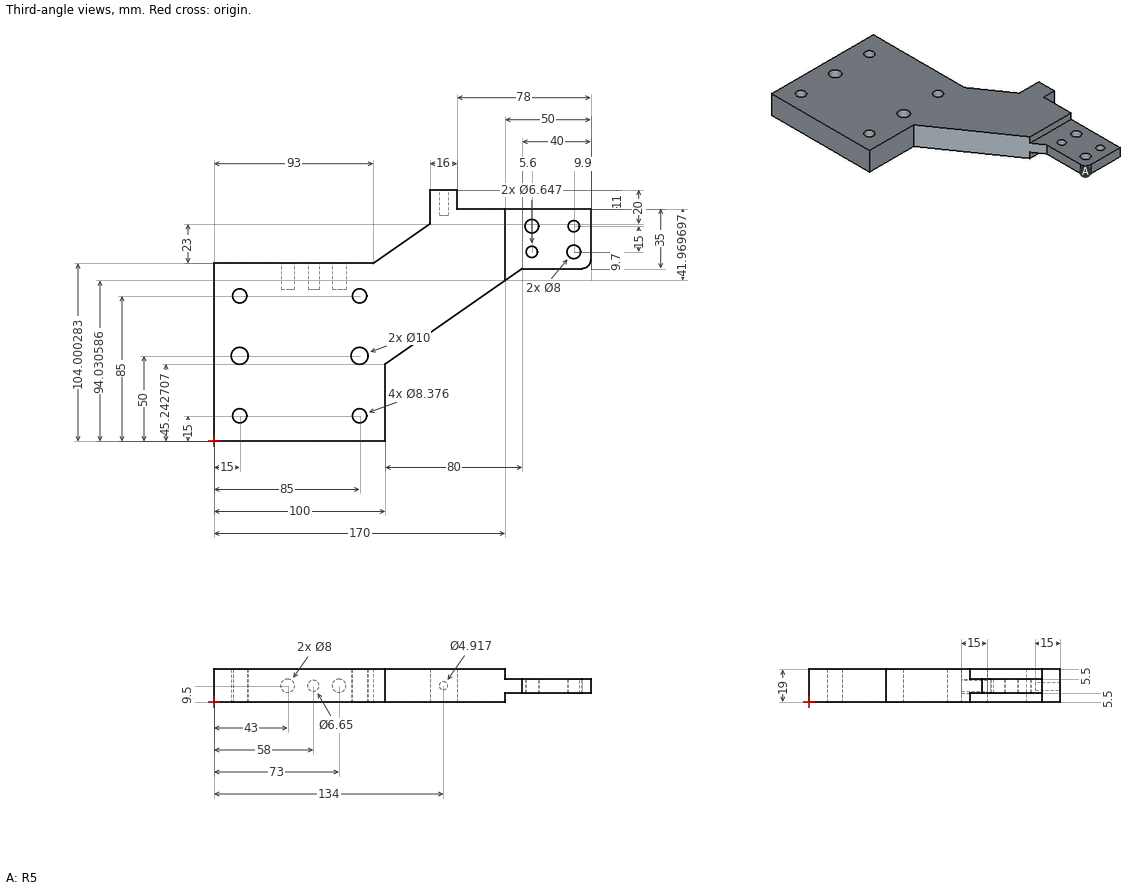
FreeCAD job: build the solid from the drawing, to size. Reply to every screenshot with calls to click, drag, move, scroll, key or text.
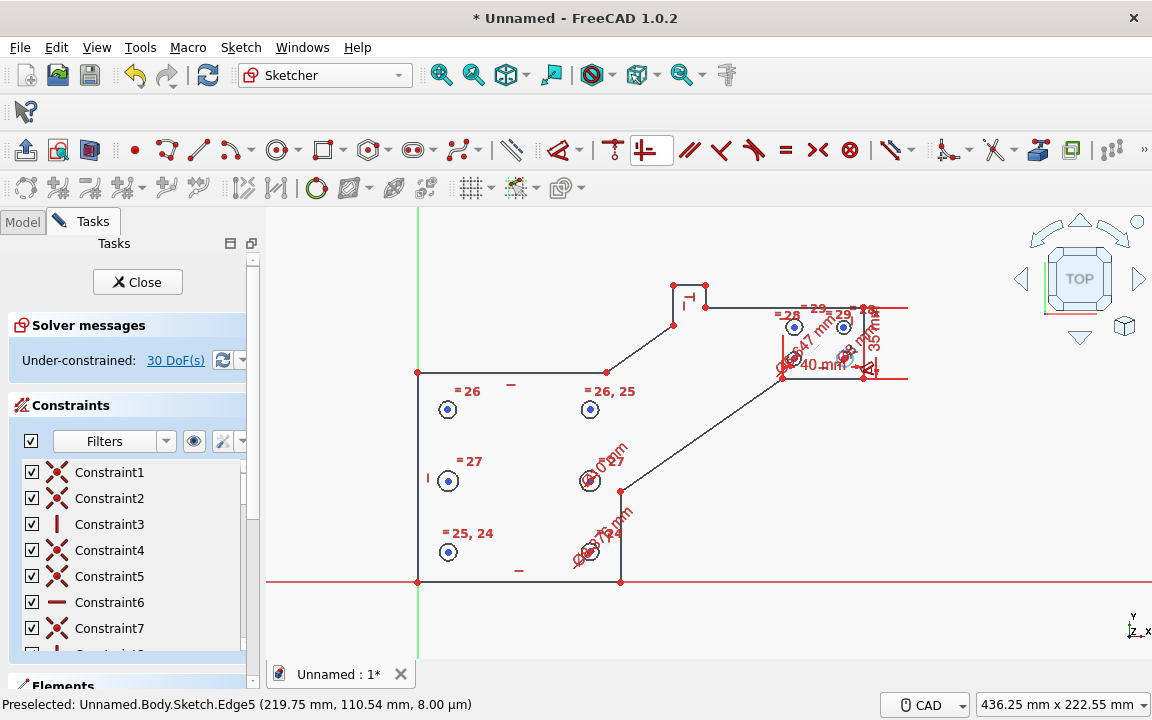
click(816, 308)
click(785, 274)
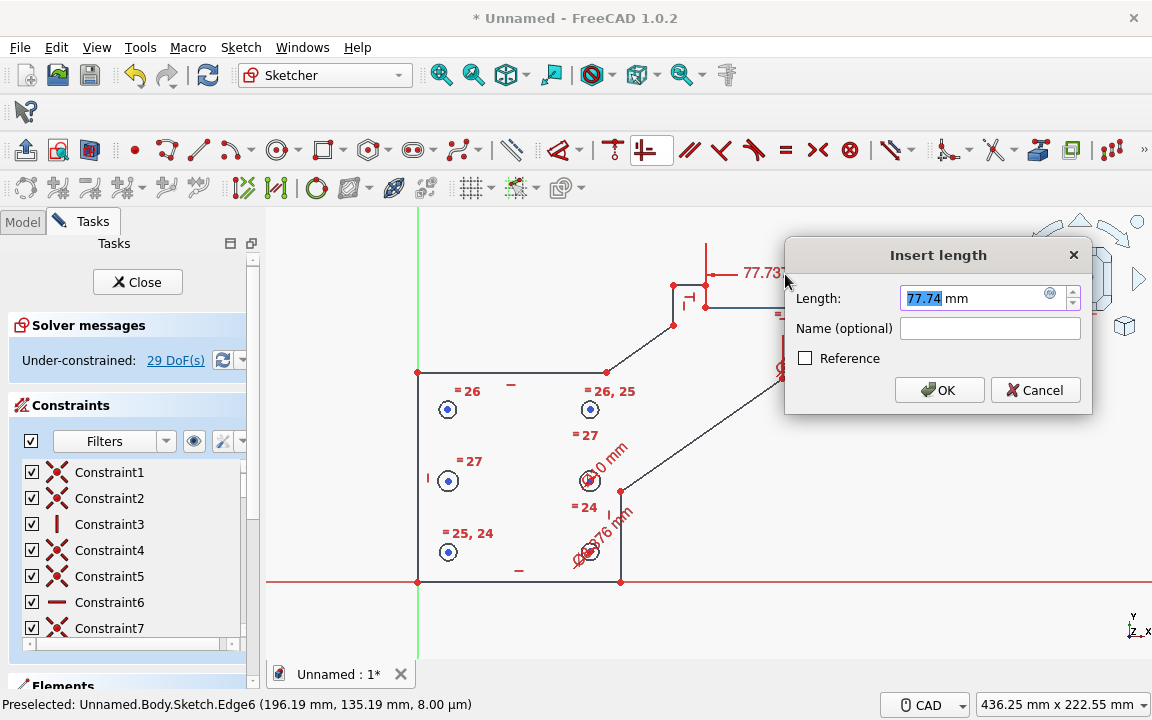
text(78)
key(Return)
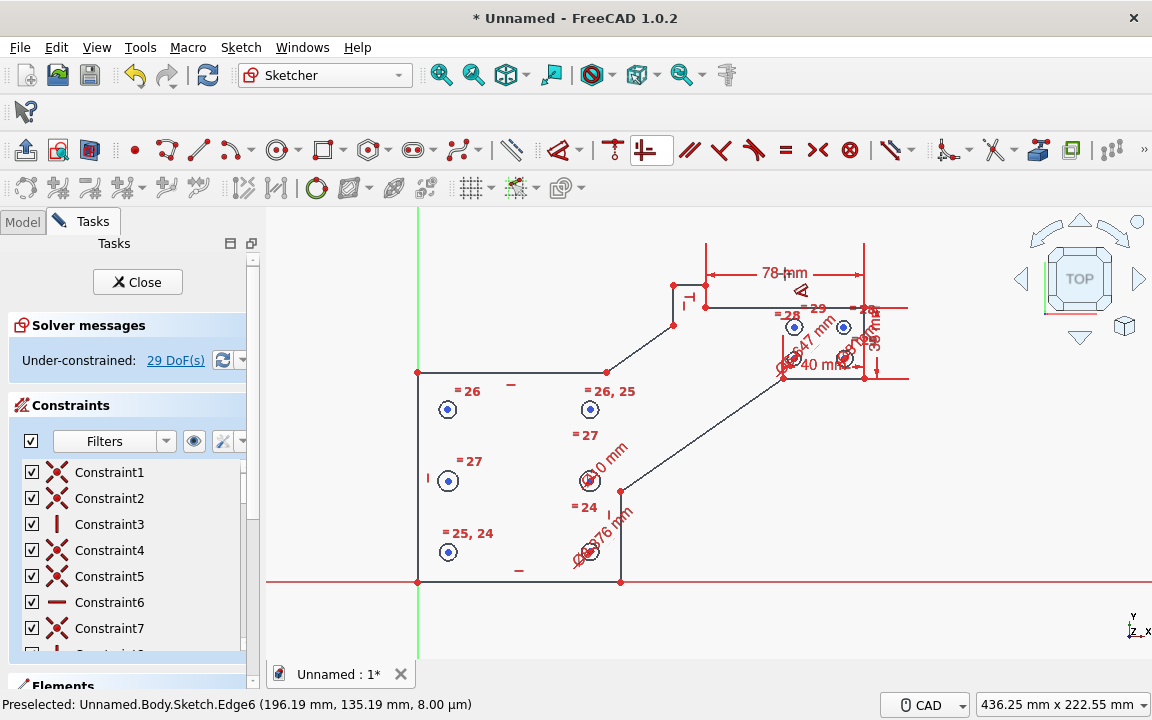
scroll(706, 296, up, 3)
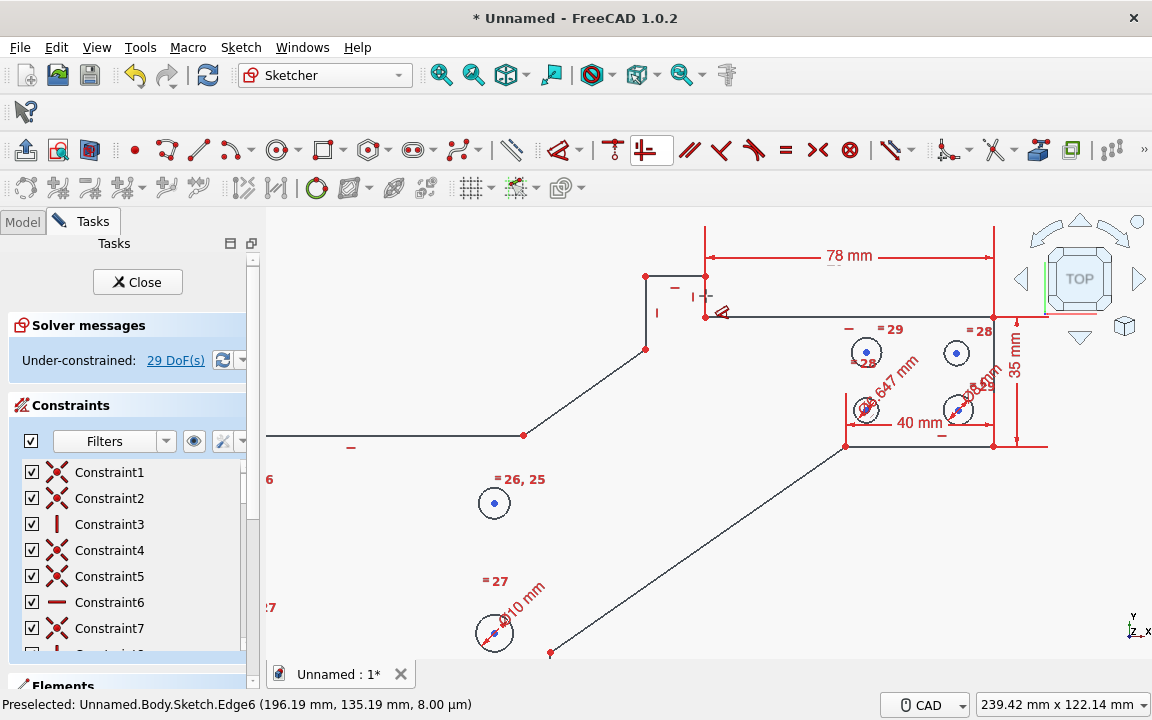
click(705, 297)
click(739, 297)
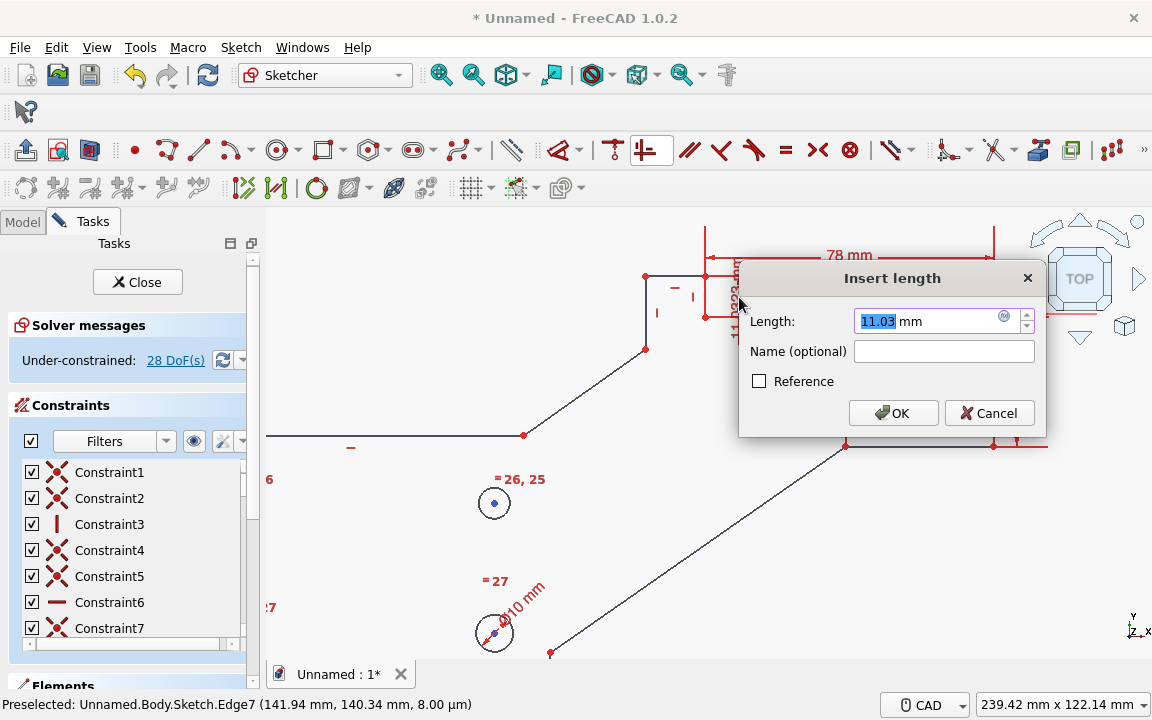
text(11)
key(Return)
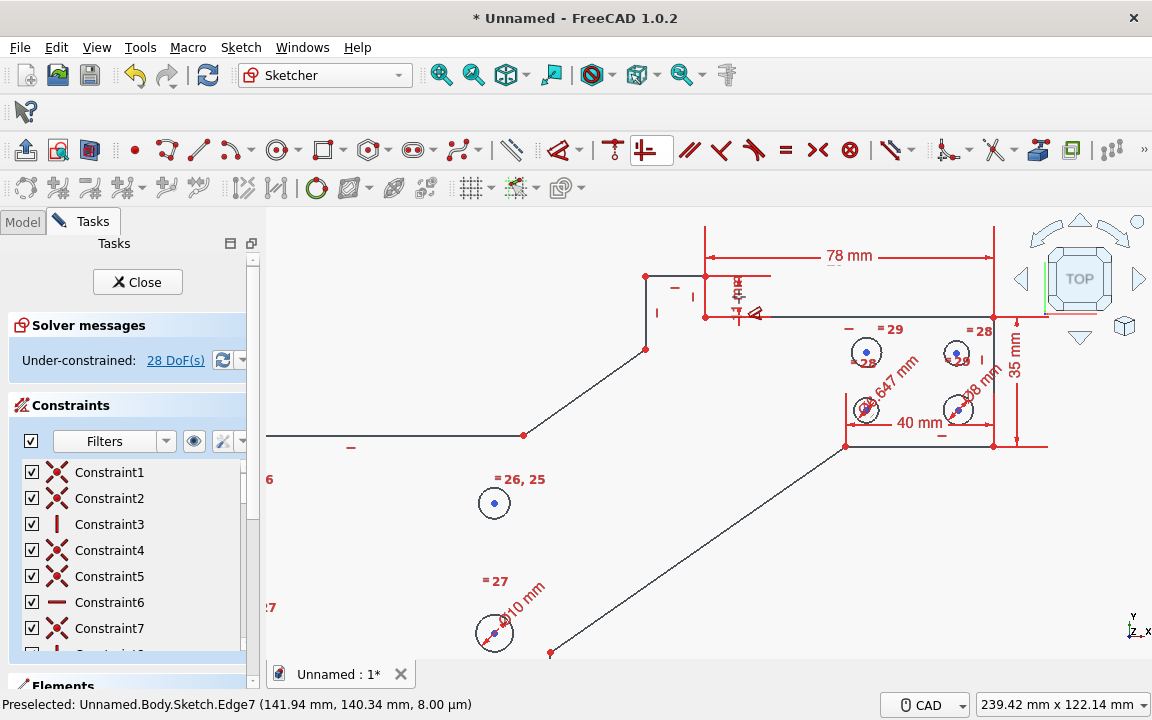
click(687, 276)
click(675, 242)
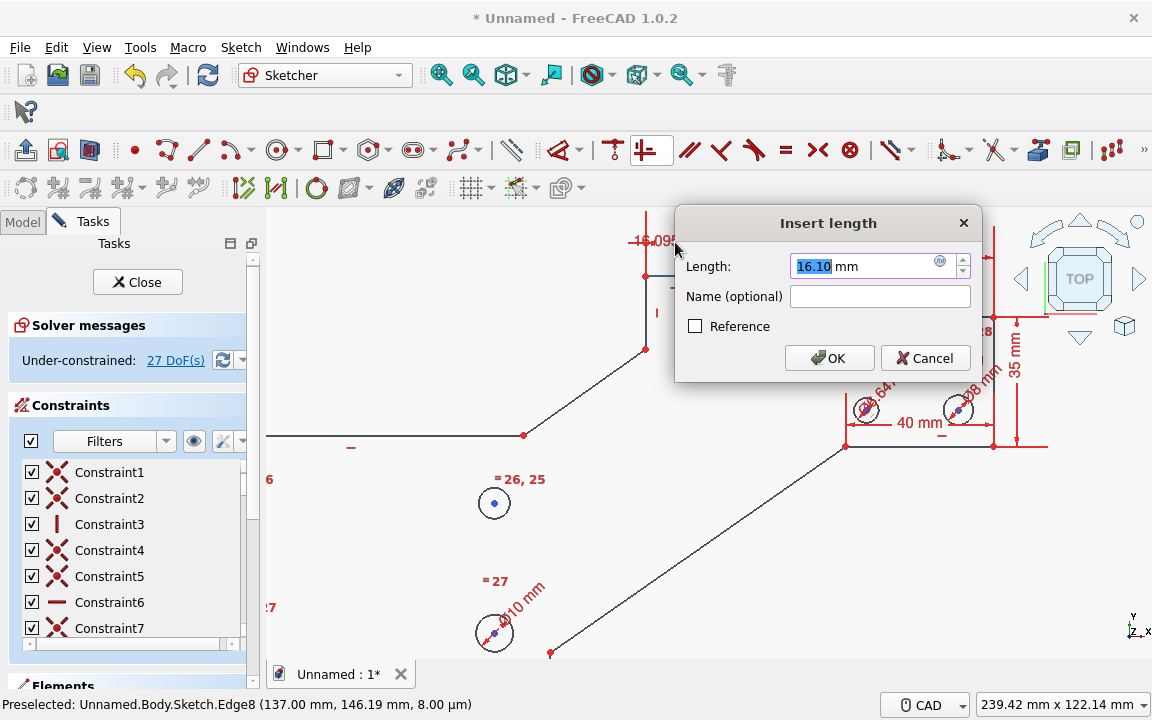
text(16)
key(Return)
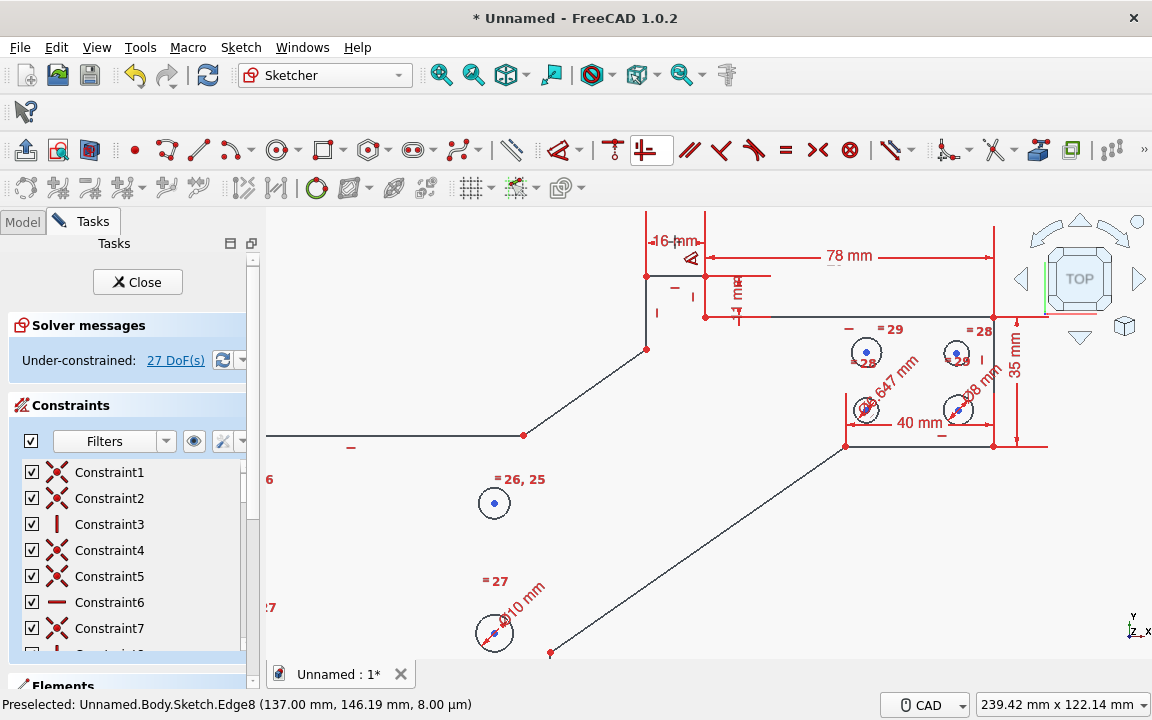
click(646, 298)
click(680, 330)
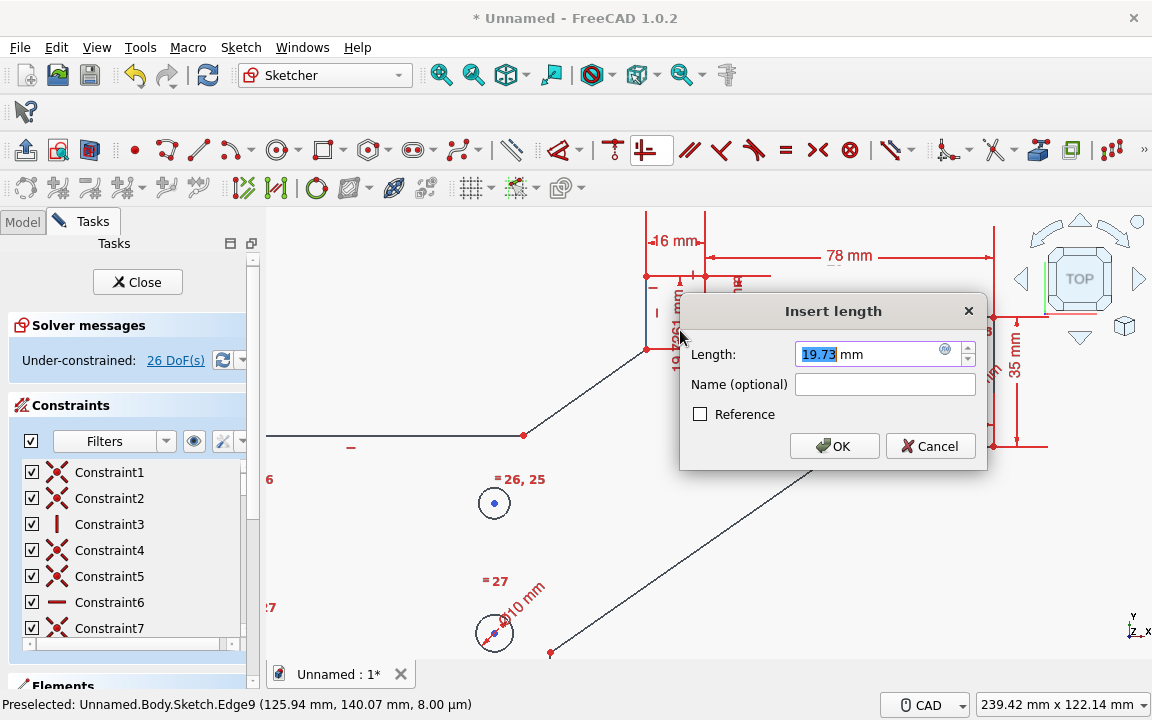
text(20)
key(Return)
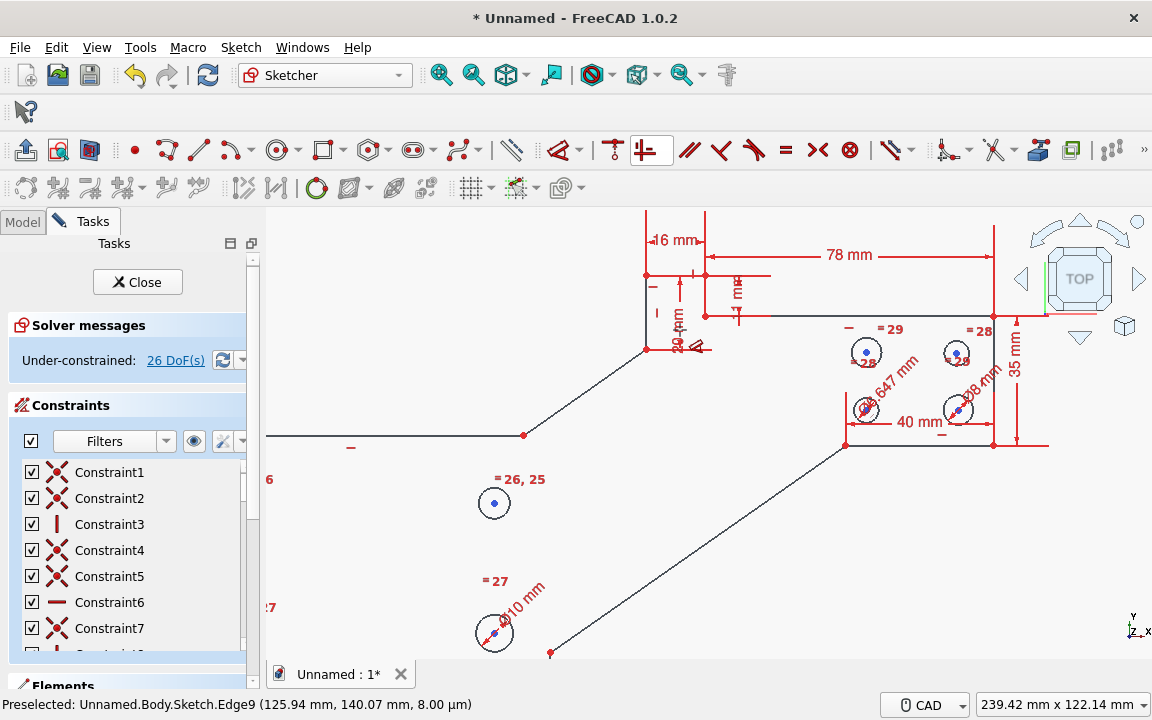
click(421, 436)
click(409, 402)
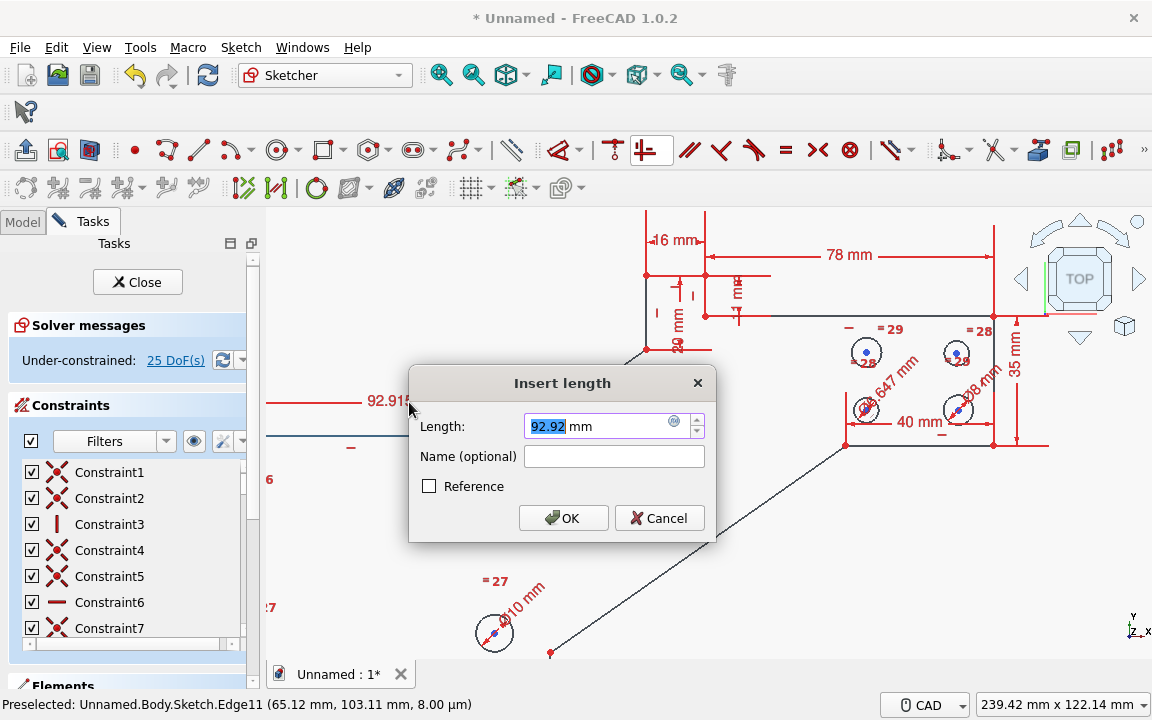
text(93)
key(Return)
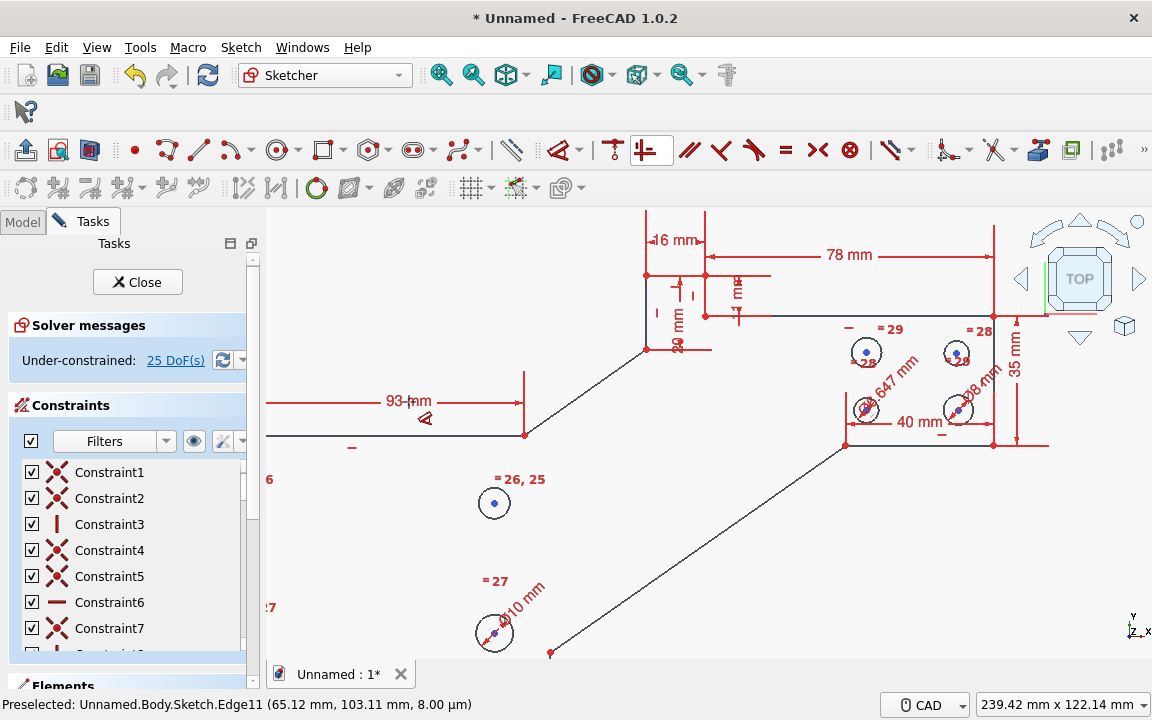
scroll(705, 296, down, 3)